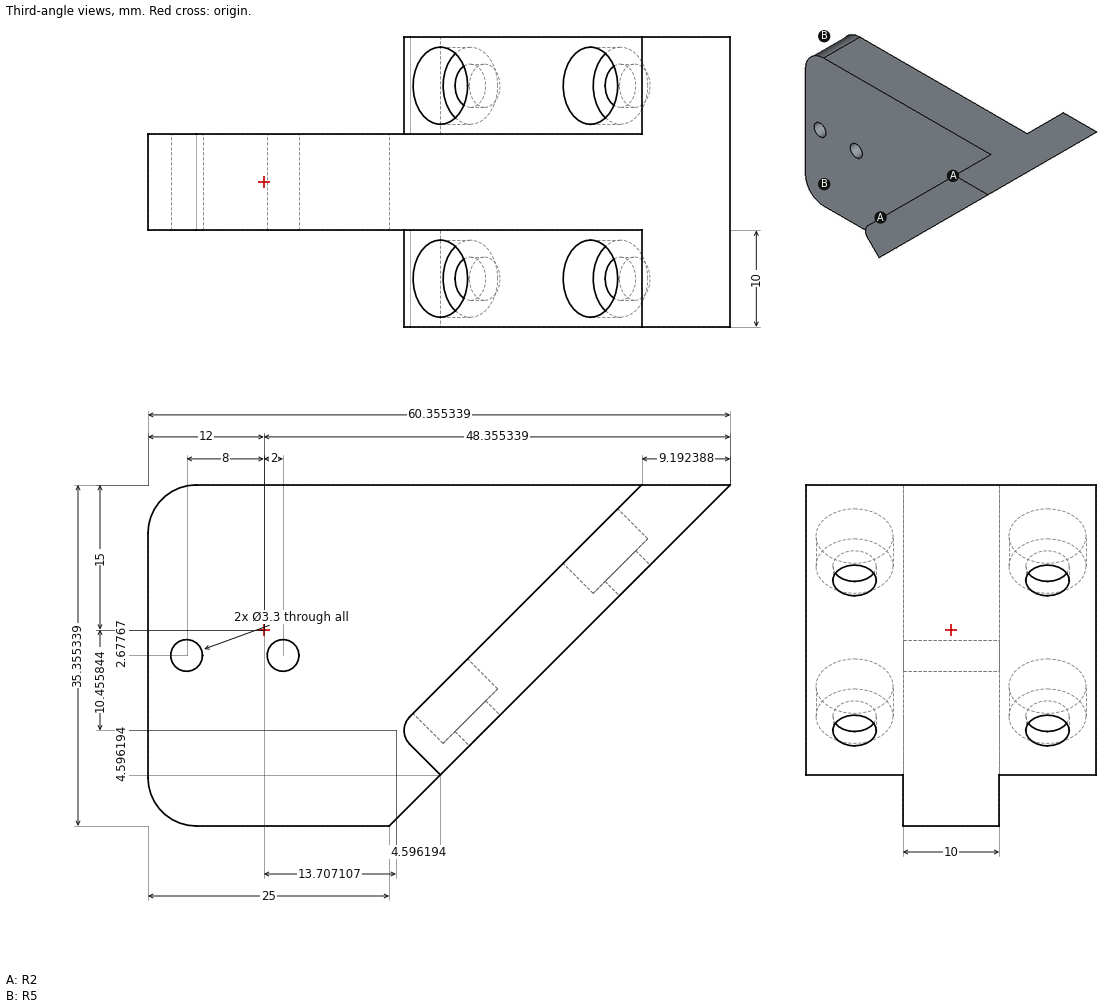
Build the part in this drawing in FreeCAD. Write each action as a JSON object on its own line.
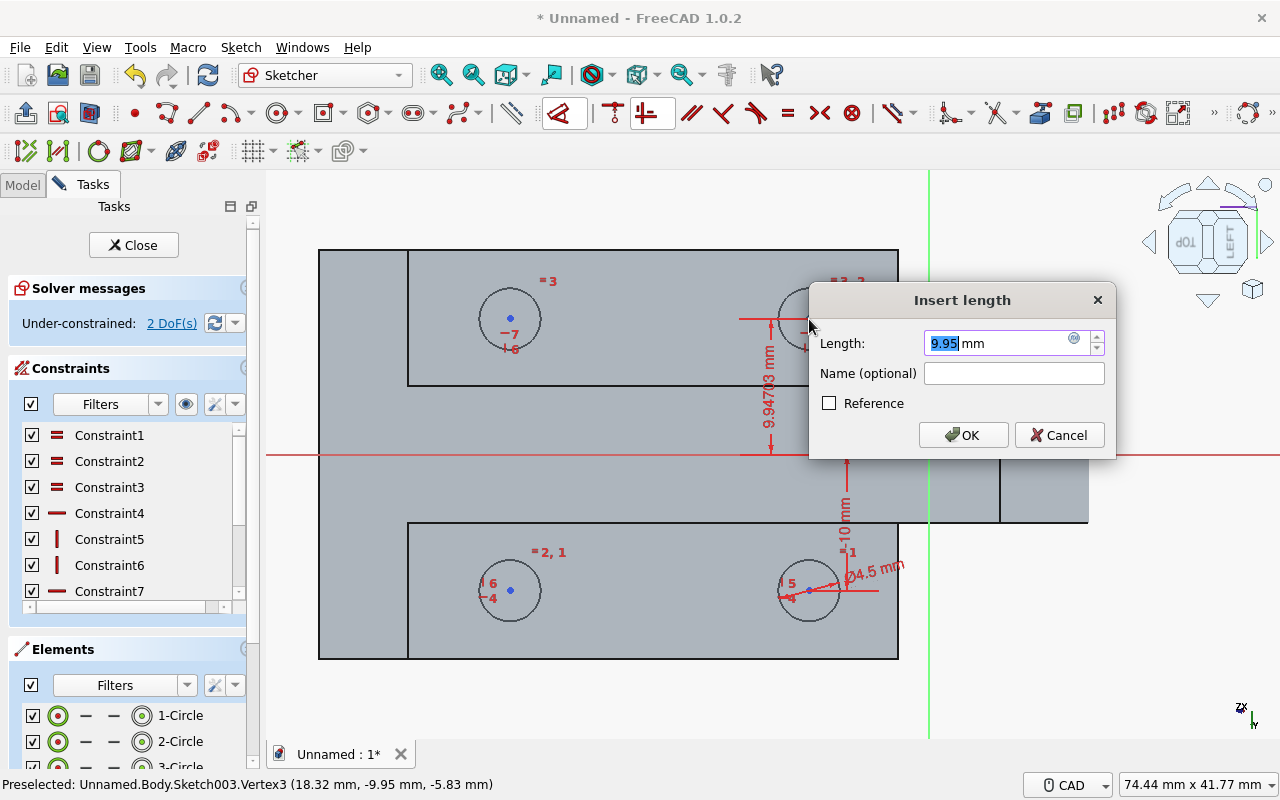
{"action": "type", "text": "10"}
{"action": "key", "text": "Return"}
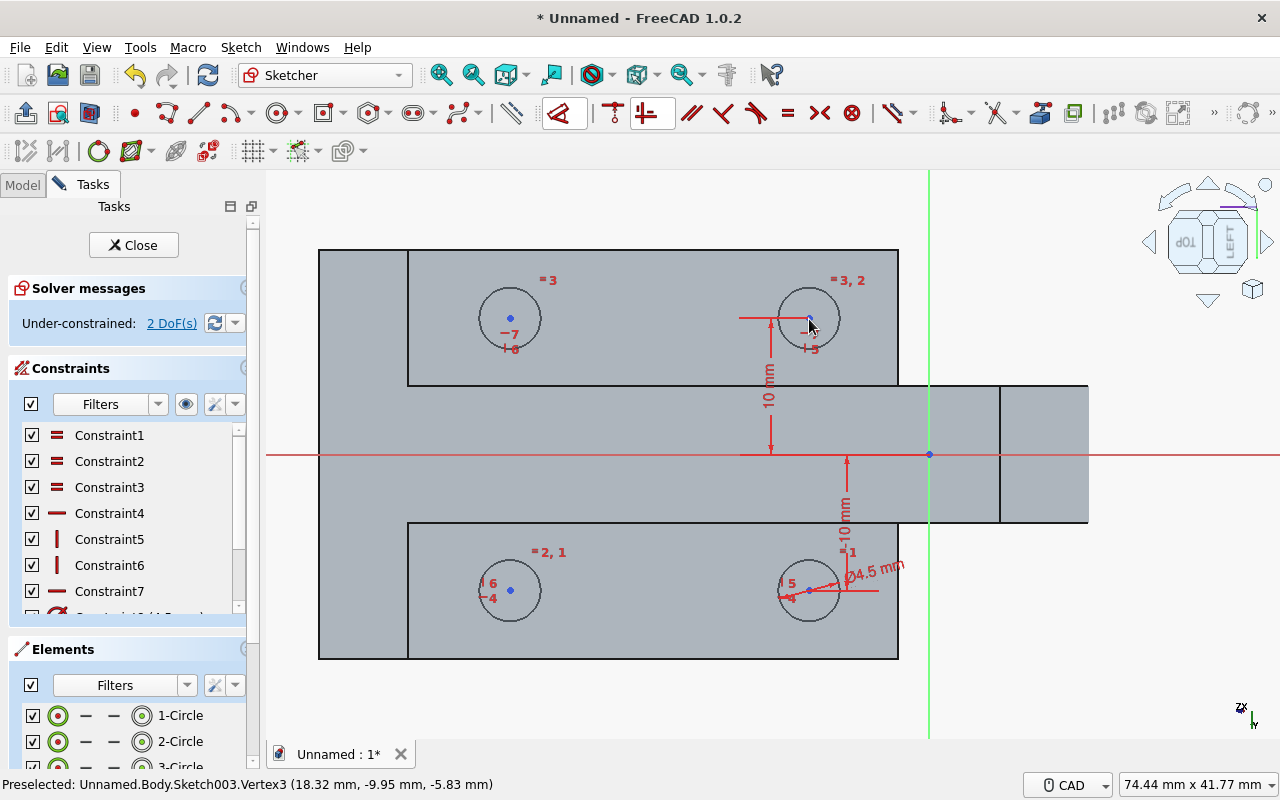
{"action": "left_click", "coordinate": [809, 591]}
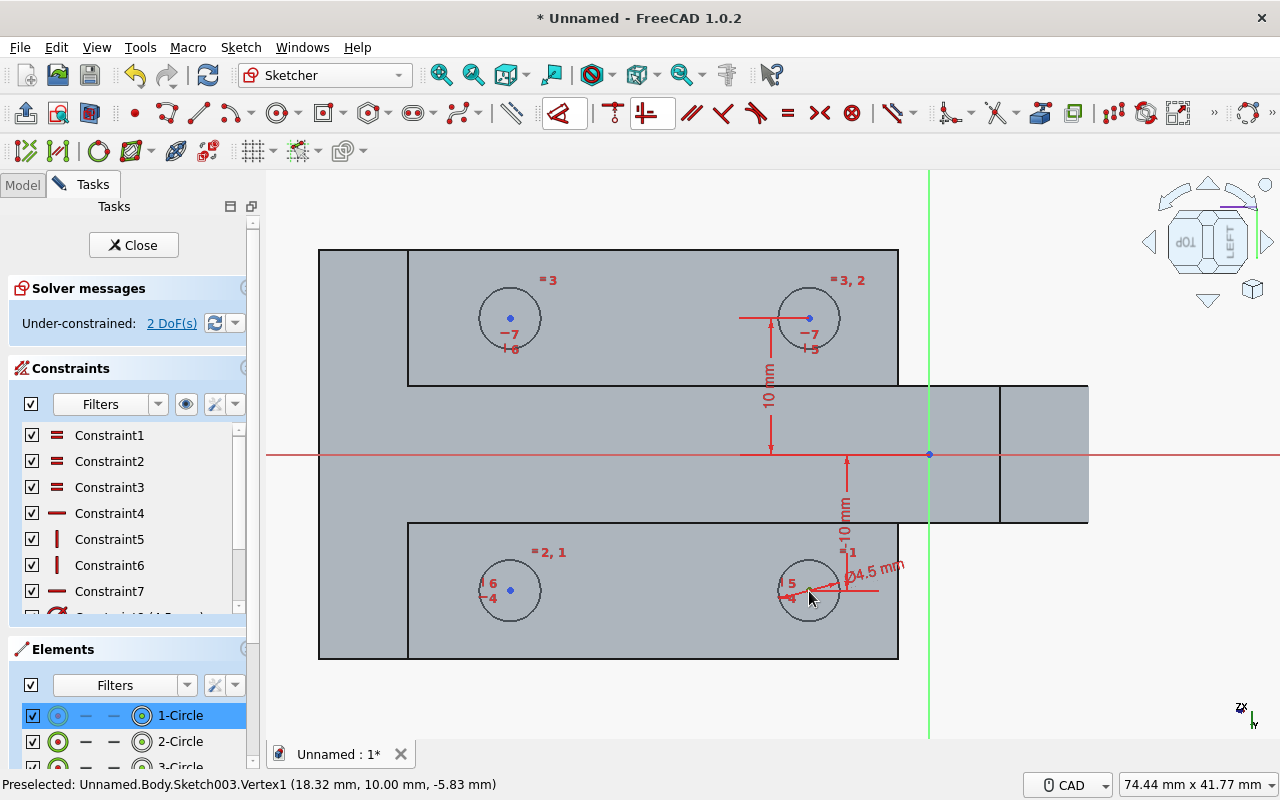
{"action": "left_click", "coordinate": [510, 591]}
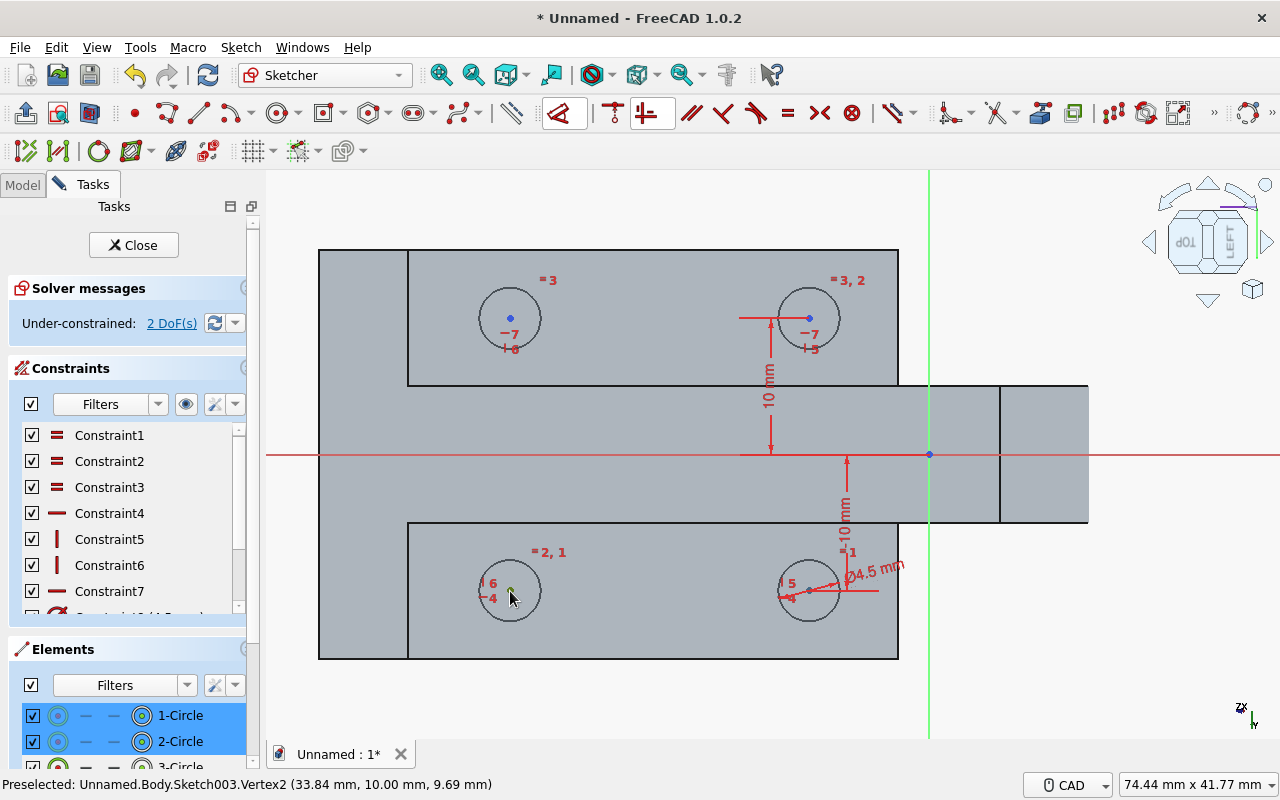
{"action": "key", "text": "l"}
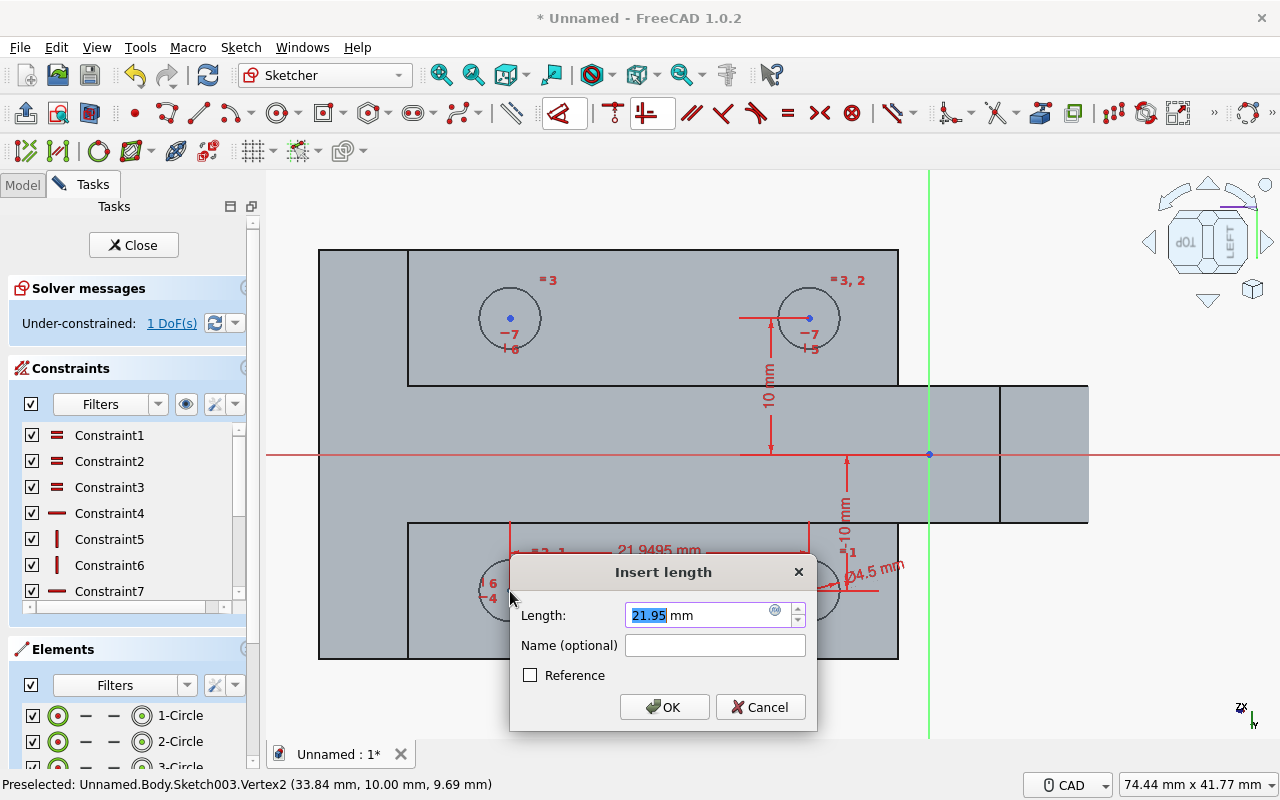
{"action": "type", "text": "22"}
{"action": "key", "text": "Return"}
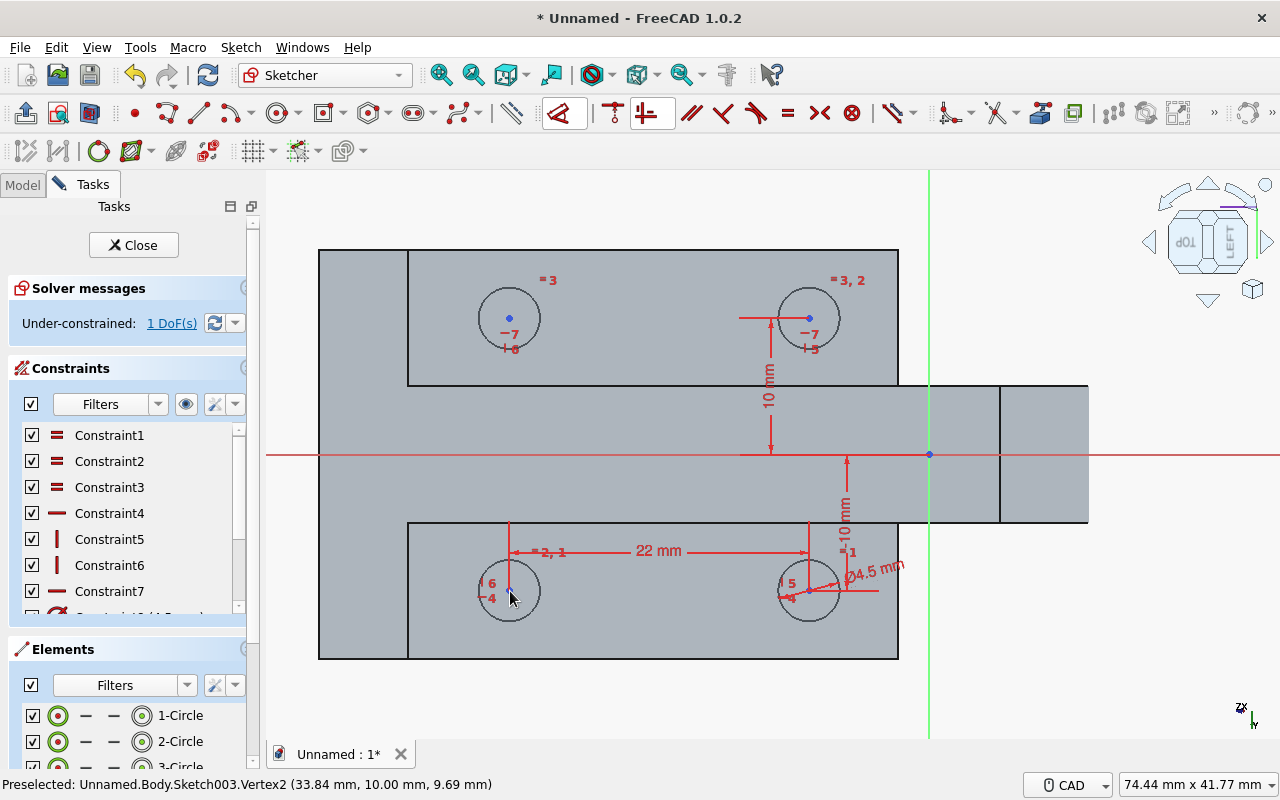
{"action": "left_click", "coordinate": [809, 591]}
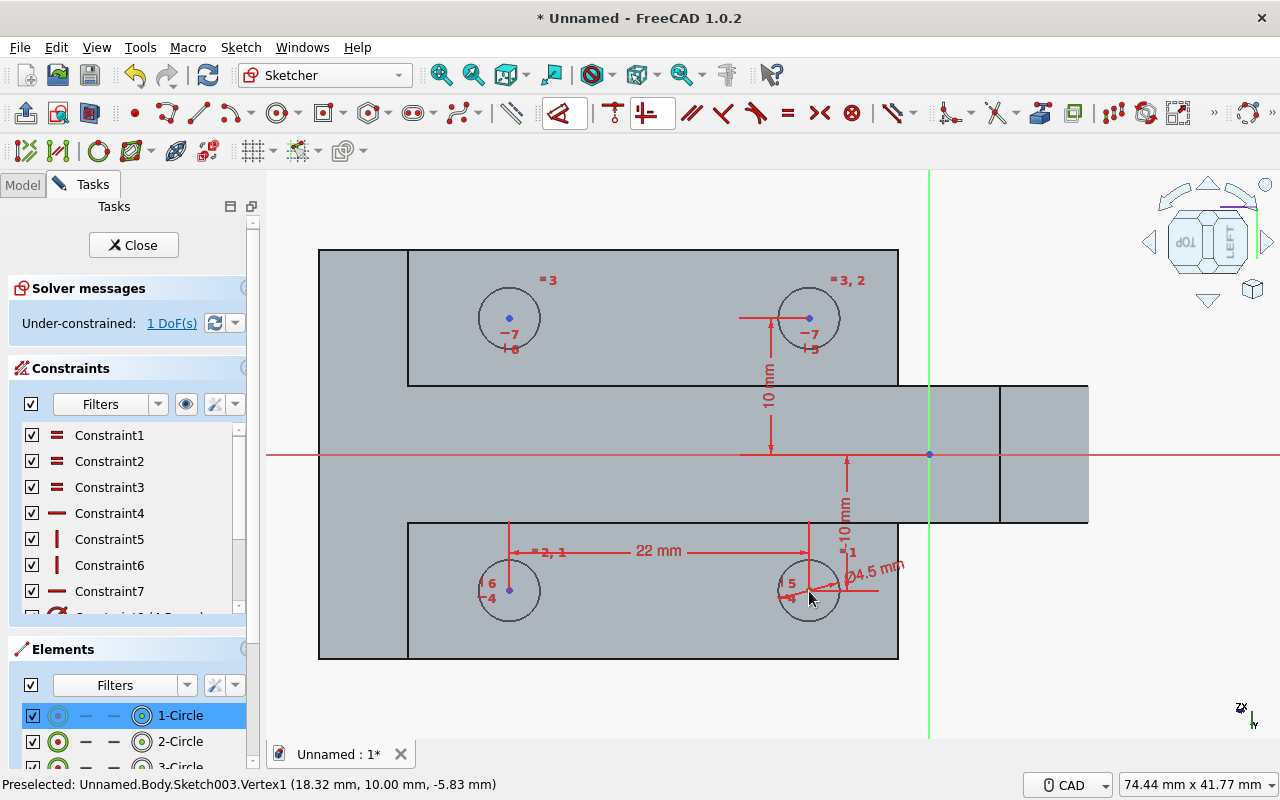
{"action": "left_click", "coordinate": [582, 114]}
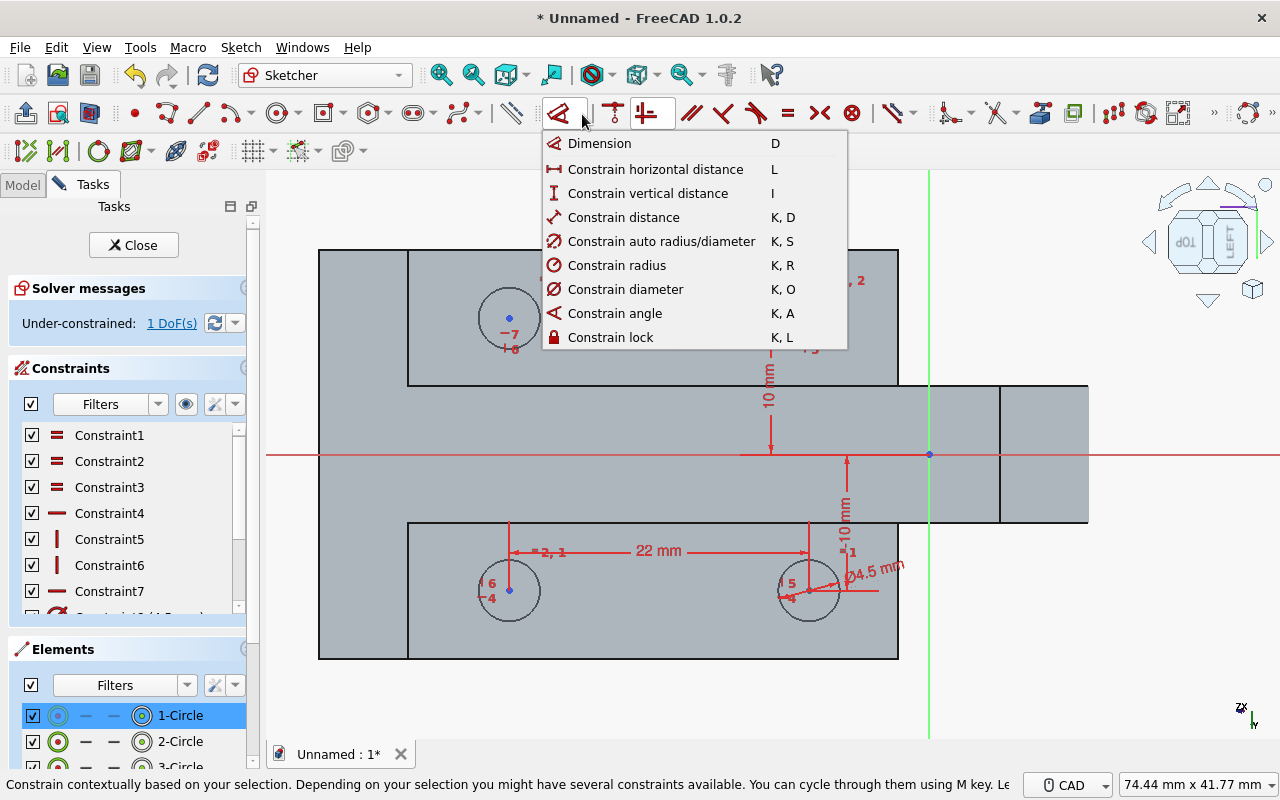
{"action": "left_click", "coordinate": [695, 169]}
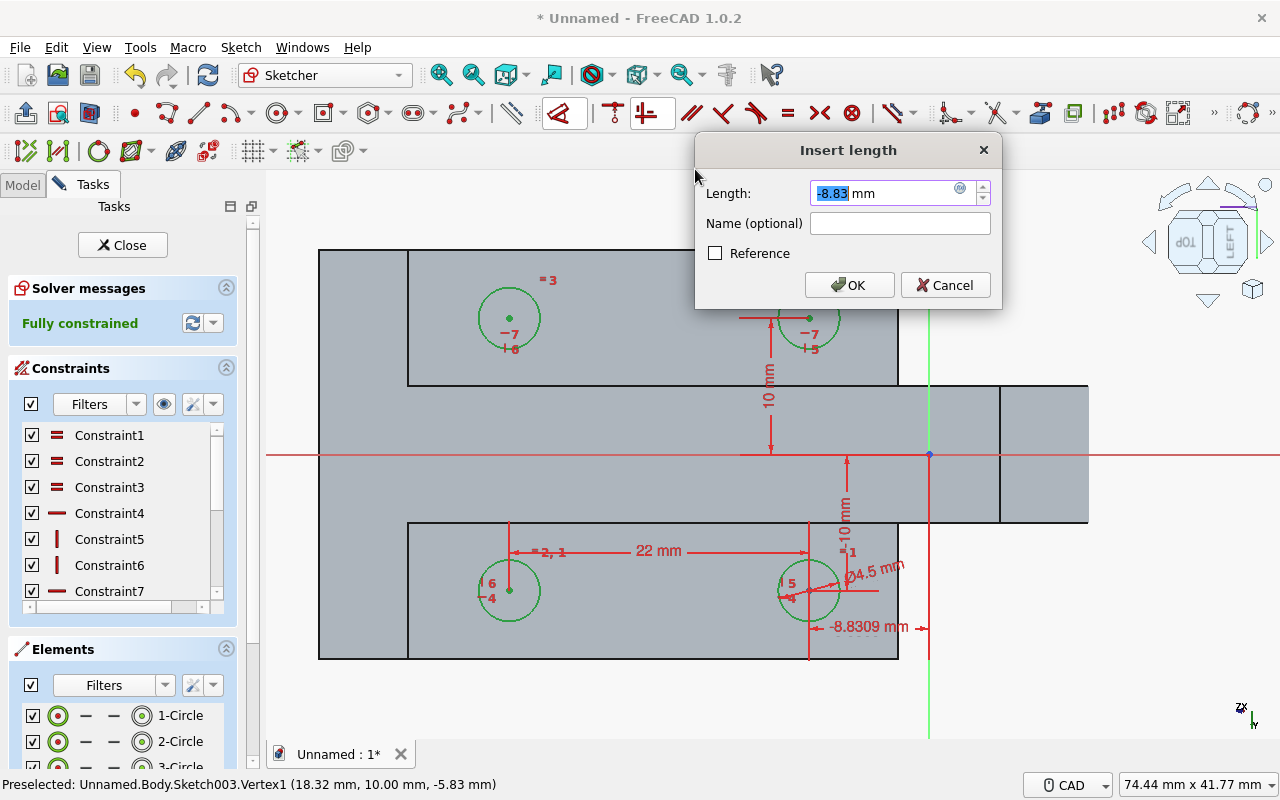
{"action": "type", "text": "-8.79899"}
{"action": "key", "text": "Return"}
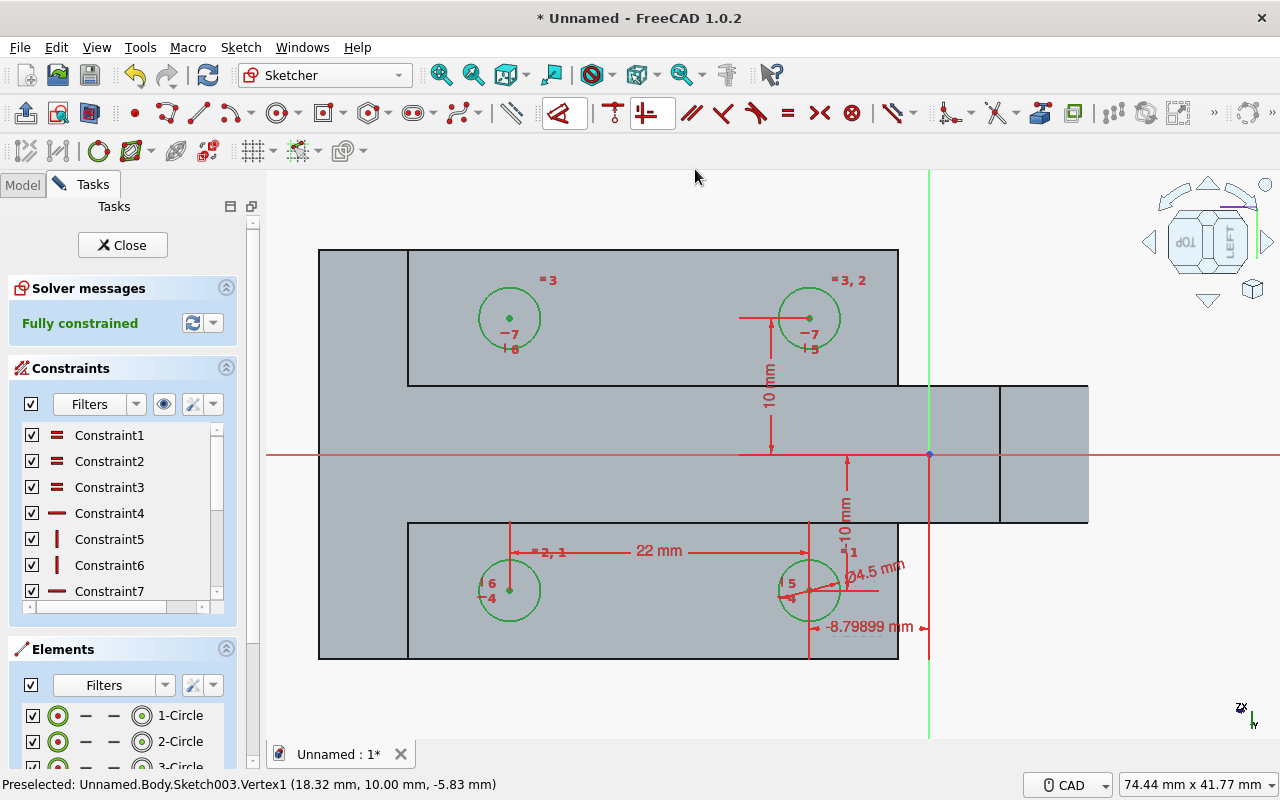
{"action": "left_click", "coordinate": [123, 245]}